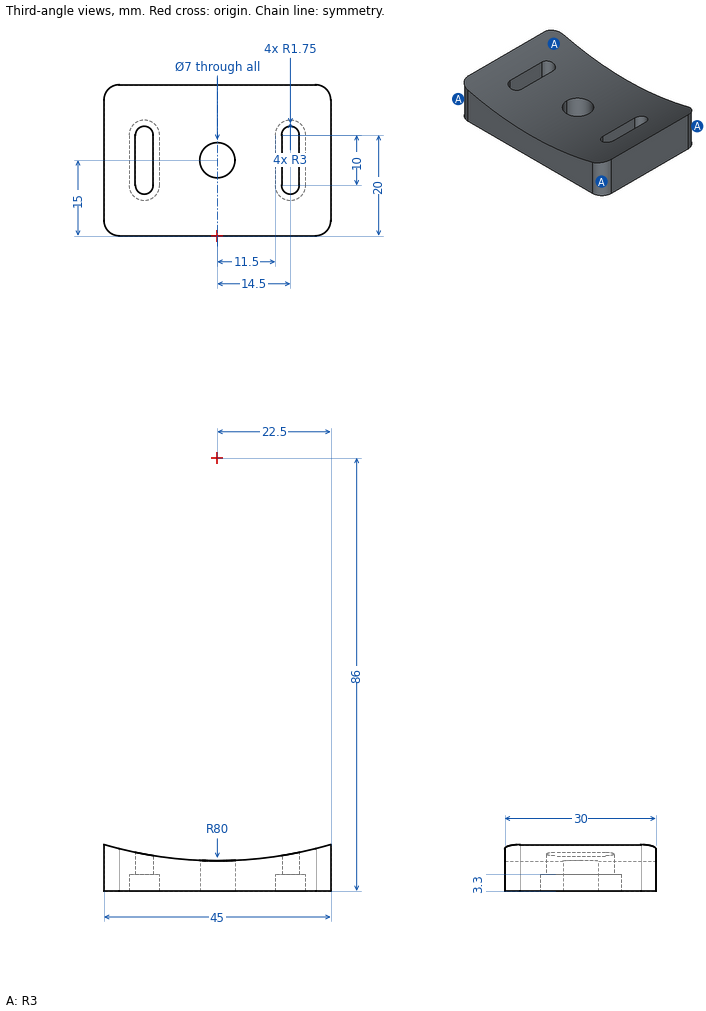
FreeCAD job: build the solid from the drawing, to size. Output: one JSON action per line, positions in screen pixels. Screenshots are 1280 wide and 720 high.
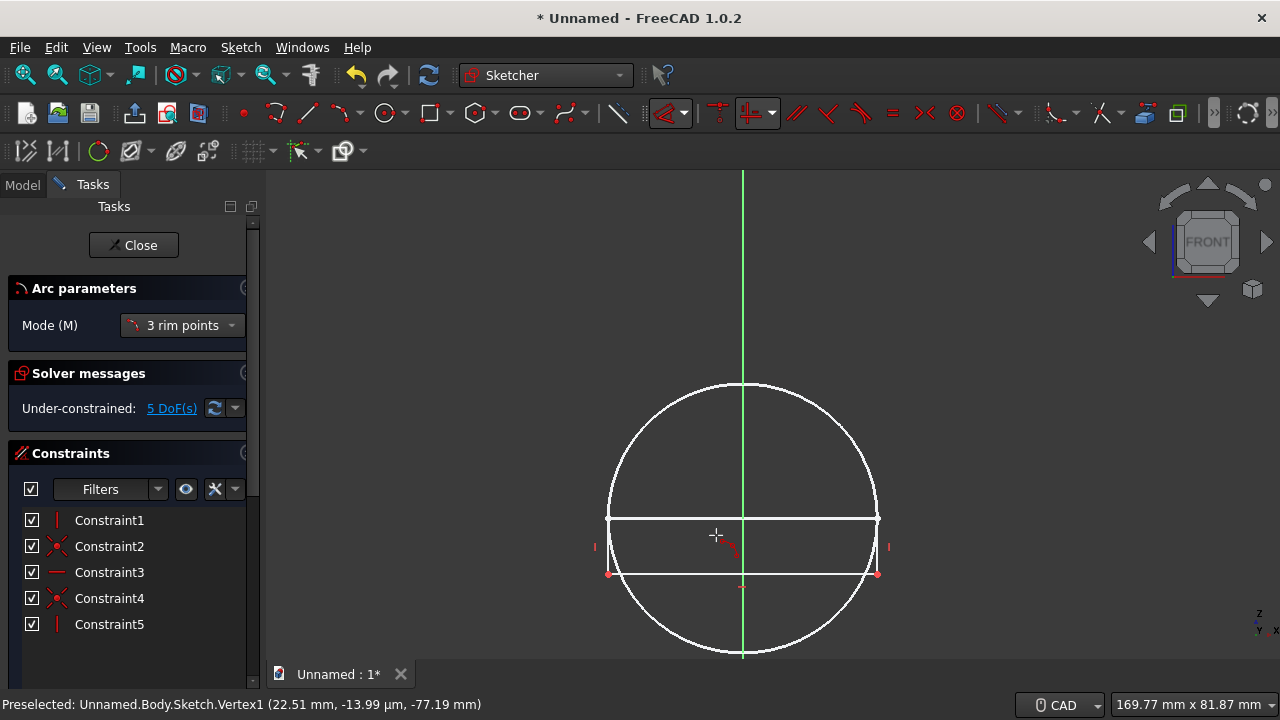
{"action": "left_click", "coordinate": [716, 534]}
{"action": "key", "text": "Escape"}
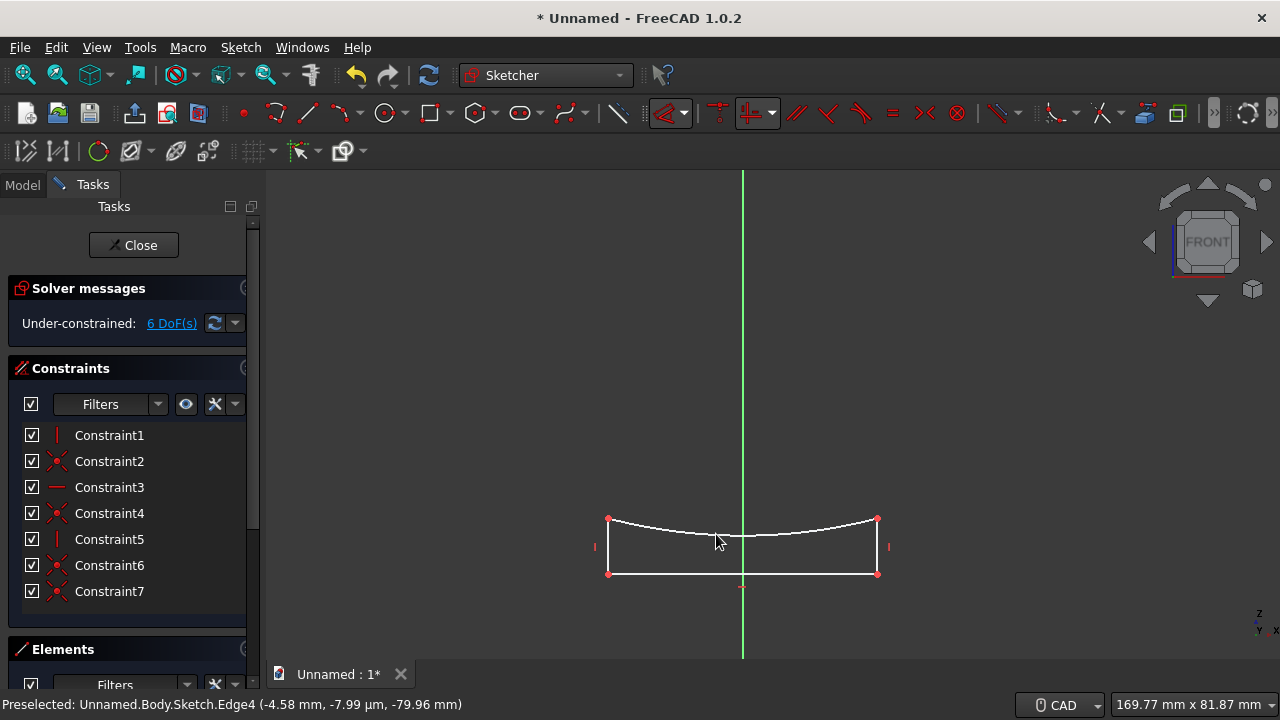
{"action": "scroll", "coordinate": [658, 536], "scroll_direction": "down", "scroll_amount": 3}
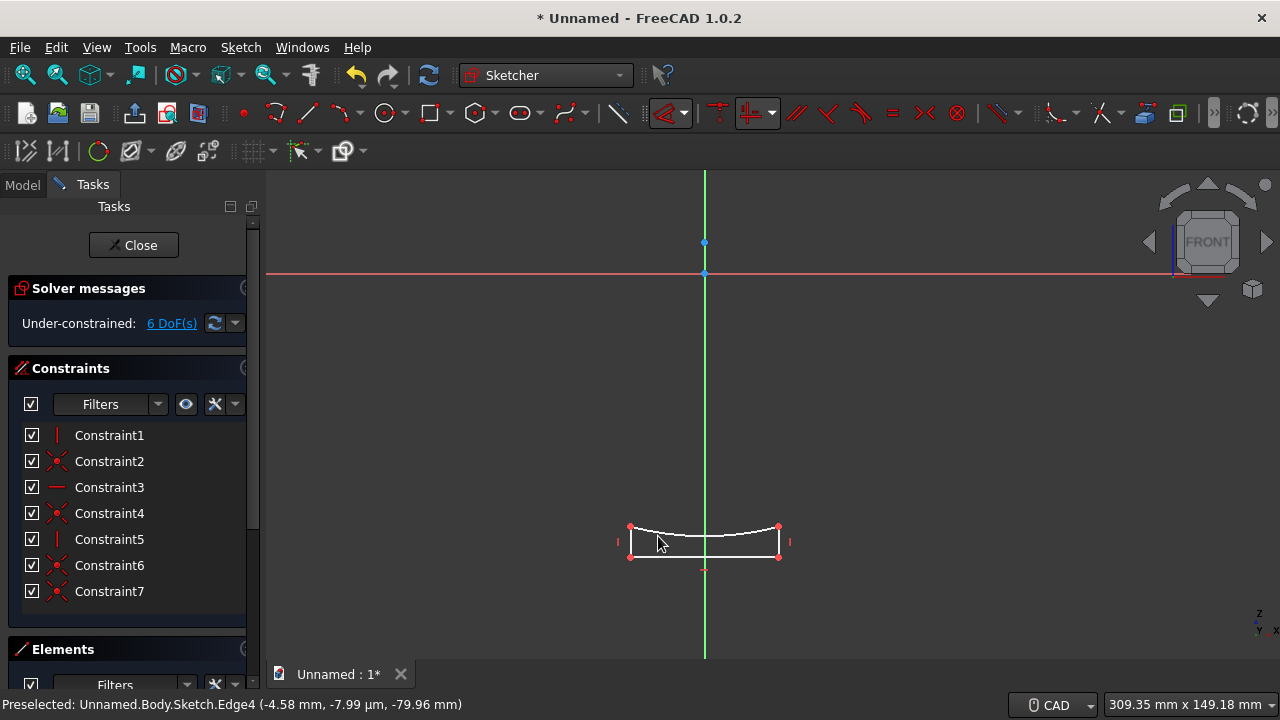
{"action": "left_click_drag", "start_coordinate": [695, 233], "coordinate": [715, 284]}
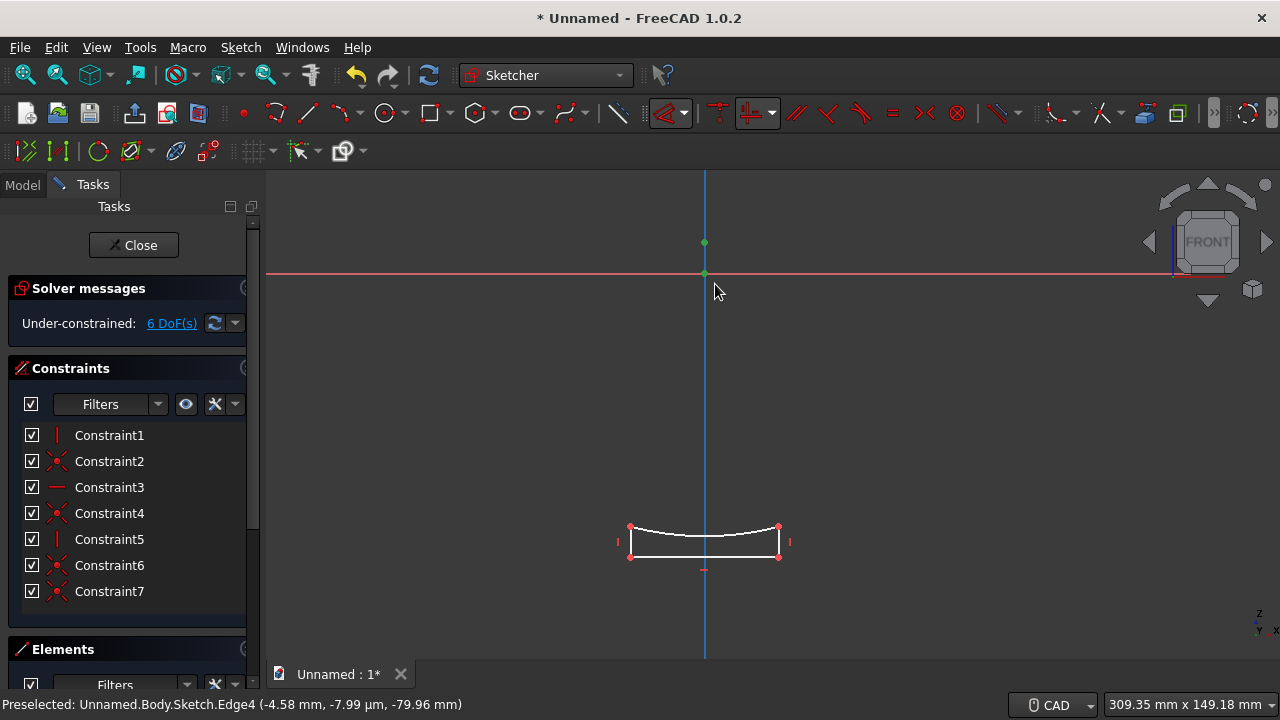
{"action": "key", "text": "c"}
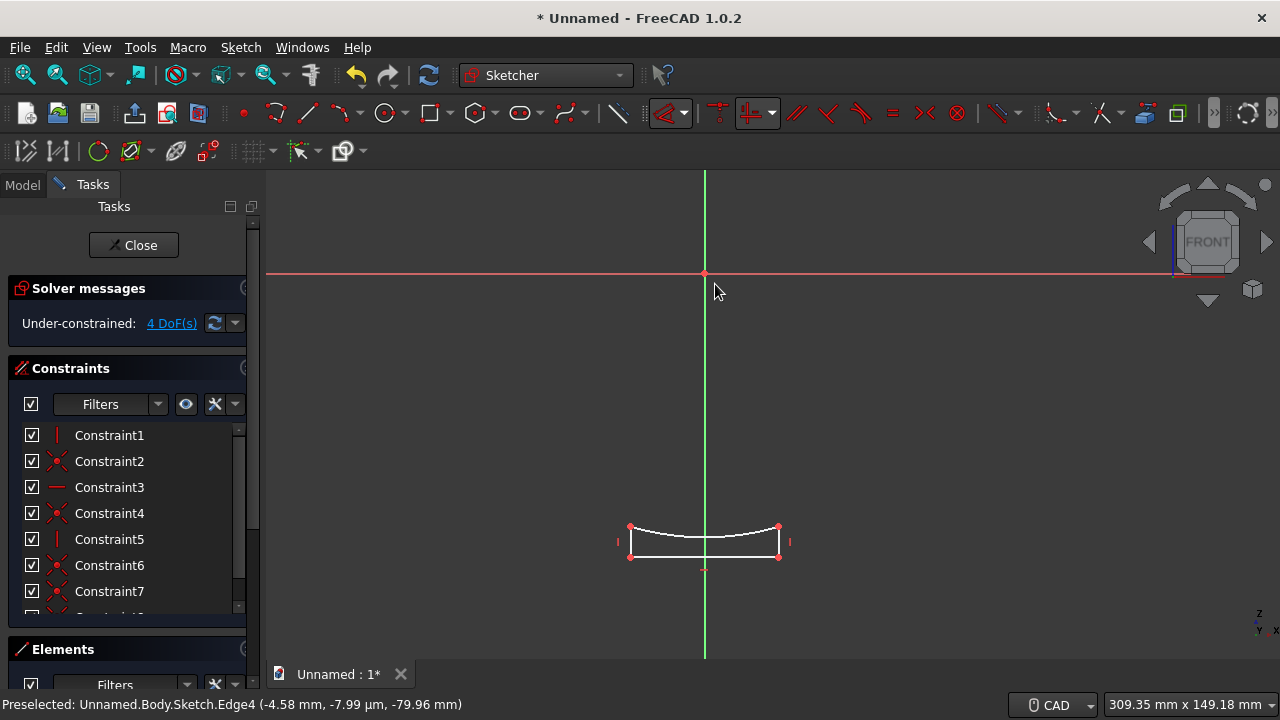
{"action": "left_click", "coordinate": [664, 114]}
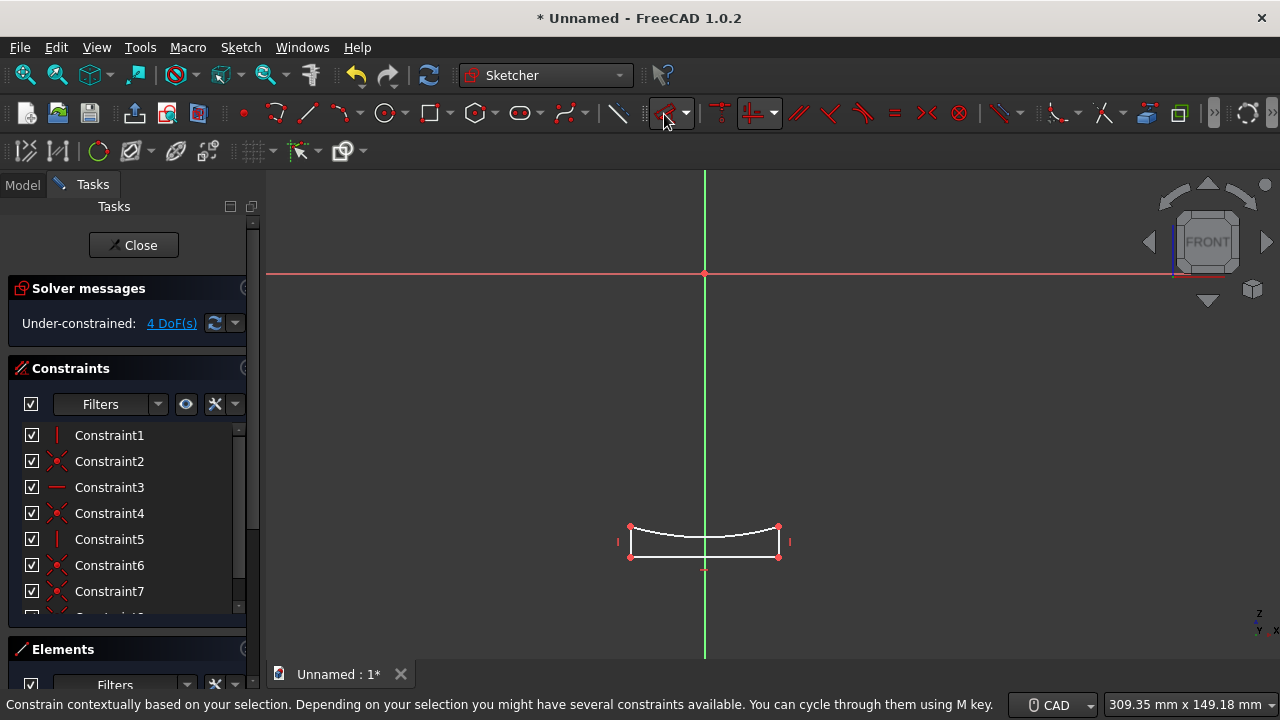
{"action": "left_click", "coordinate": [675, 536]}
{"action": "left_click", "coordinate": [534, 516]}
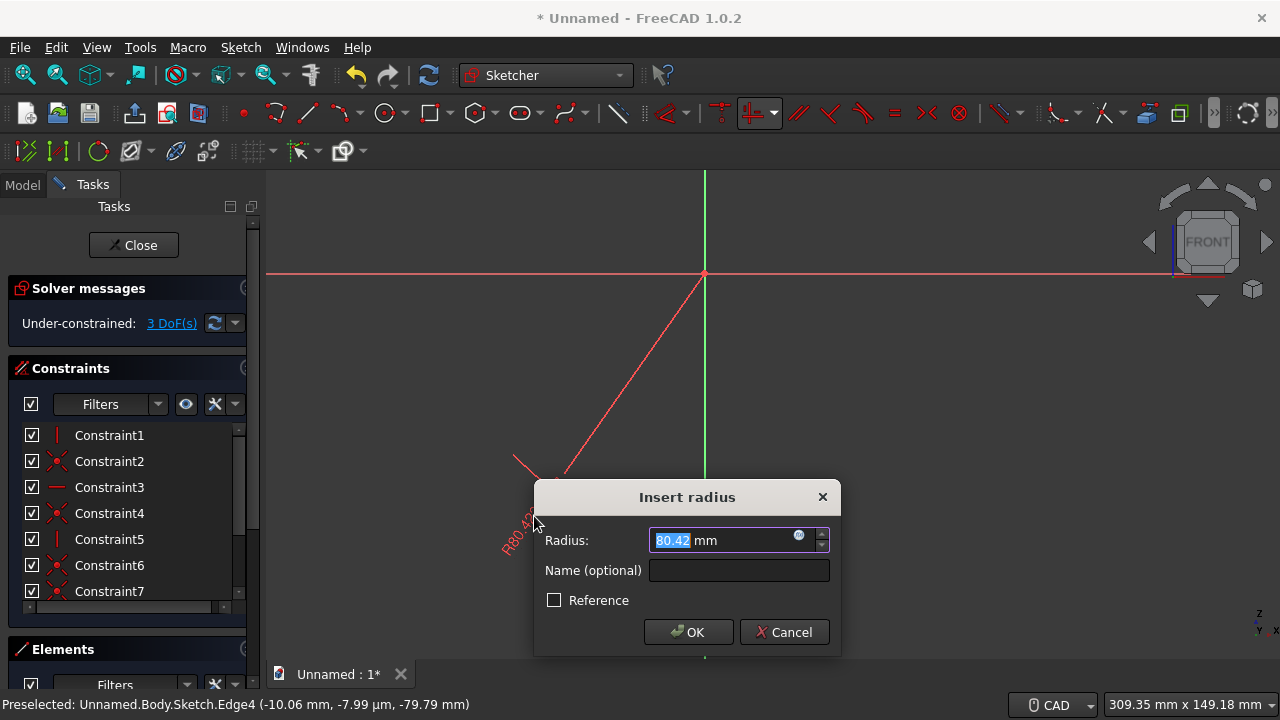
{"action": "type", "text": "80"}
{"action": "key", "text": "Return"}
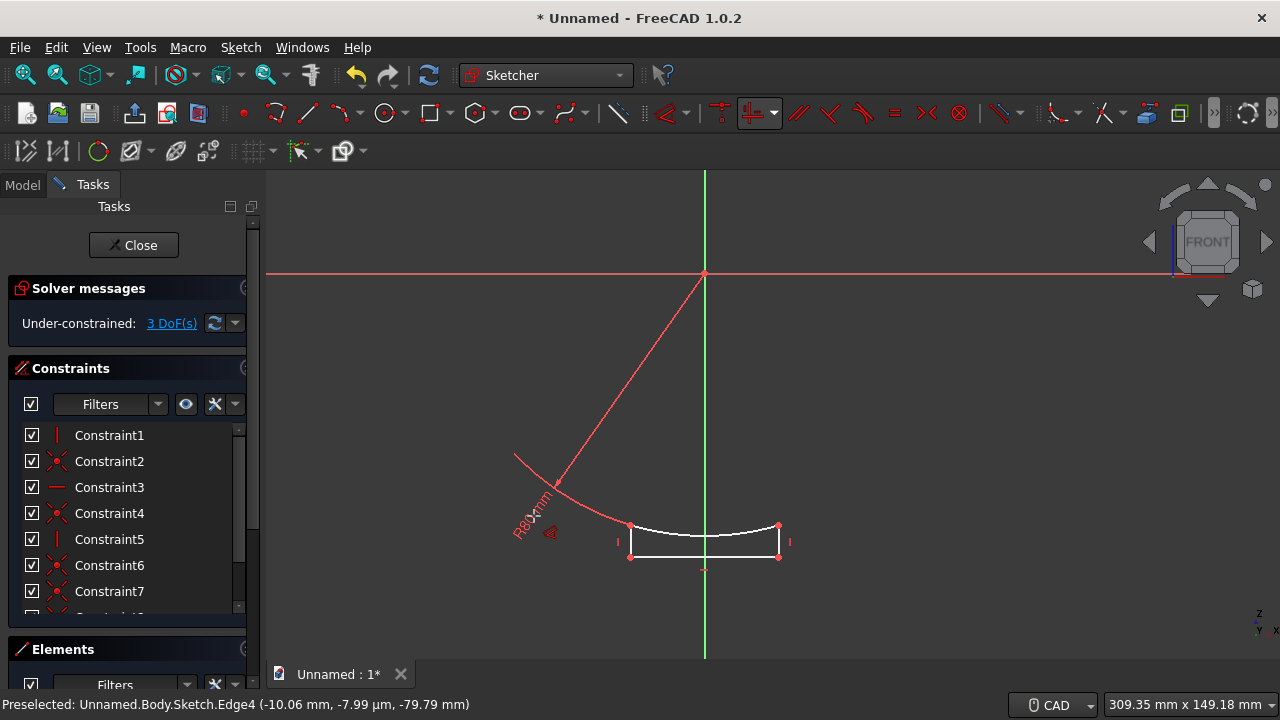
{"action": "left_click", "coordinate": [734, 557]}
{"action": "left_click", "coordinate": [671, 591]}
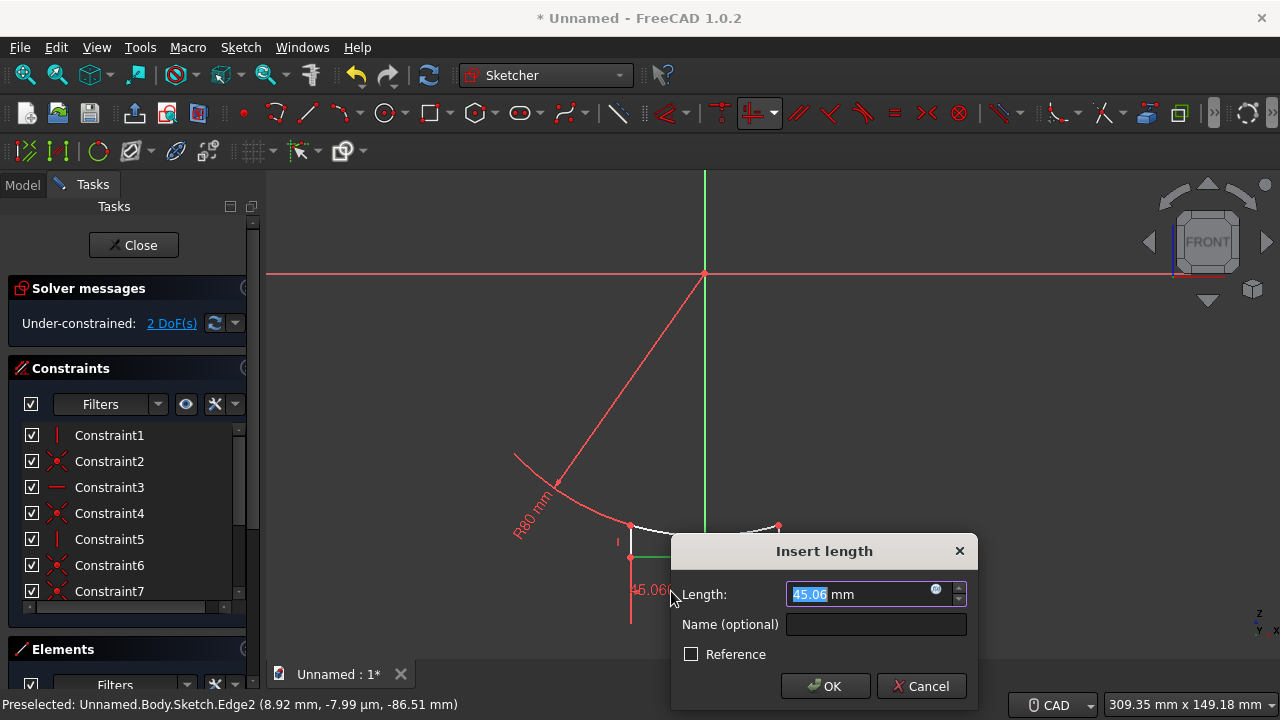
{"action": "type", "text": "45"}
{"action": "key", "text": "Return"}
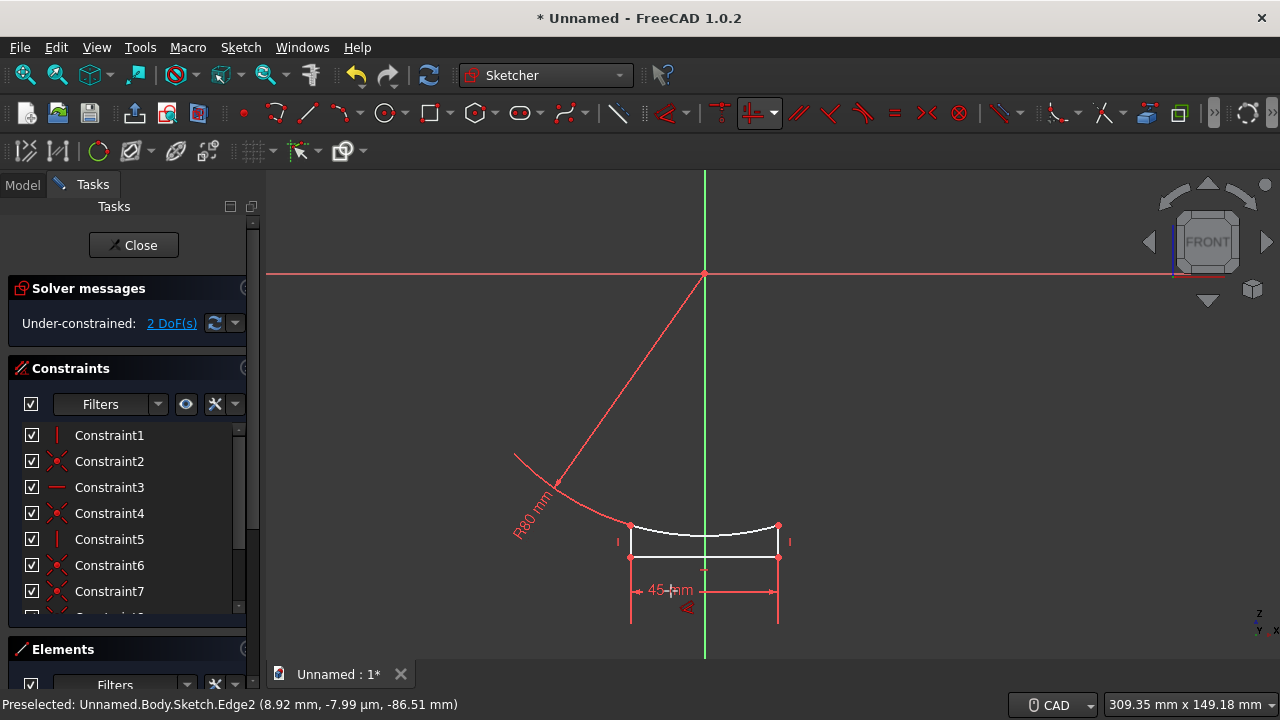
{"action": "left_click", "coordinate": [778, 557]}
{"action": "left_click", "coordinate": [812, 415]}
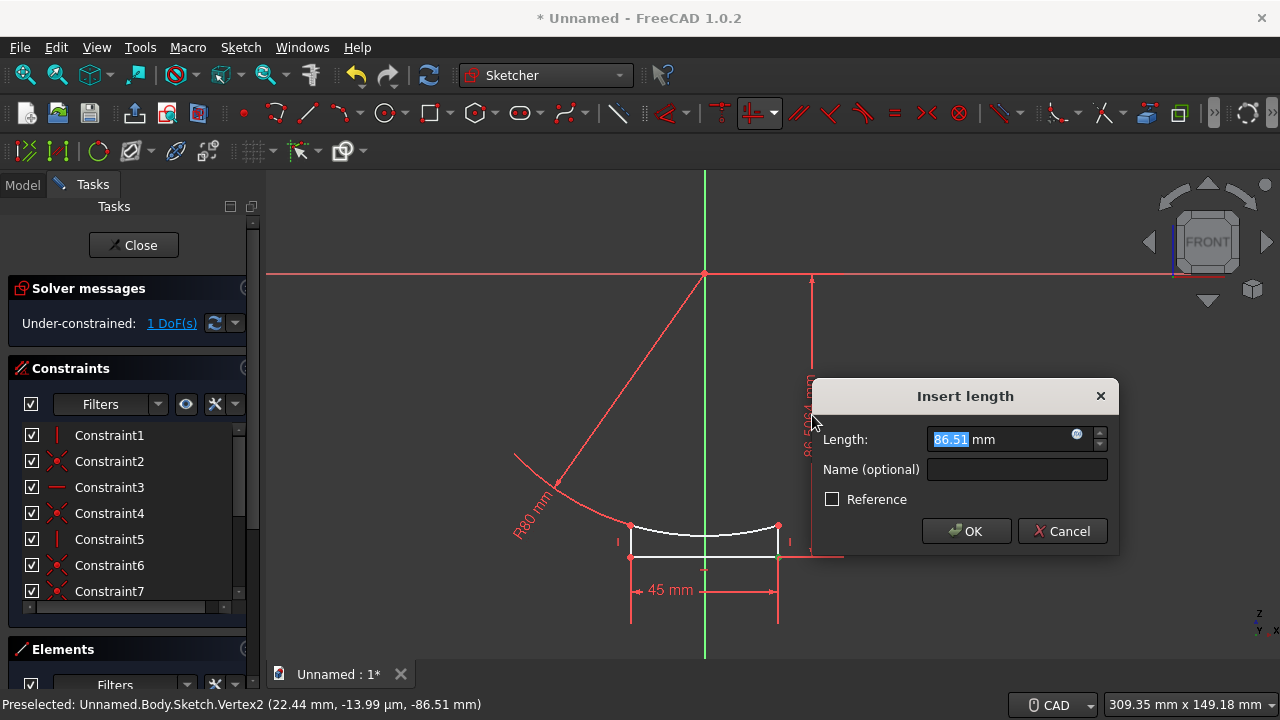
{"action": "type", "text": "86"}
{"action": "key", "text": "Return"}